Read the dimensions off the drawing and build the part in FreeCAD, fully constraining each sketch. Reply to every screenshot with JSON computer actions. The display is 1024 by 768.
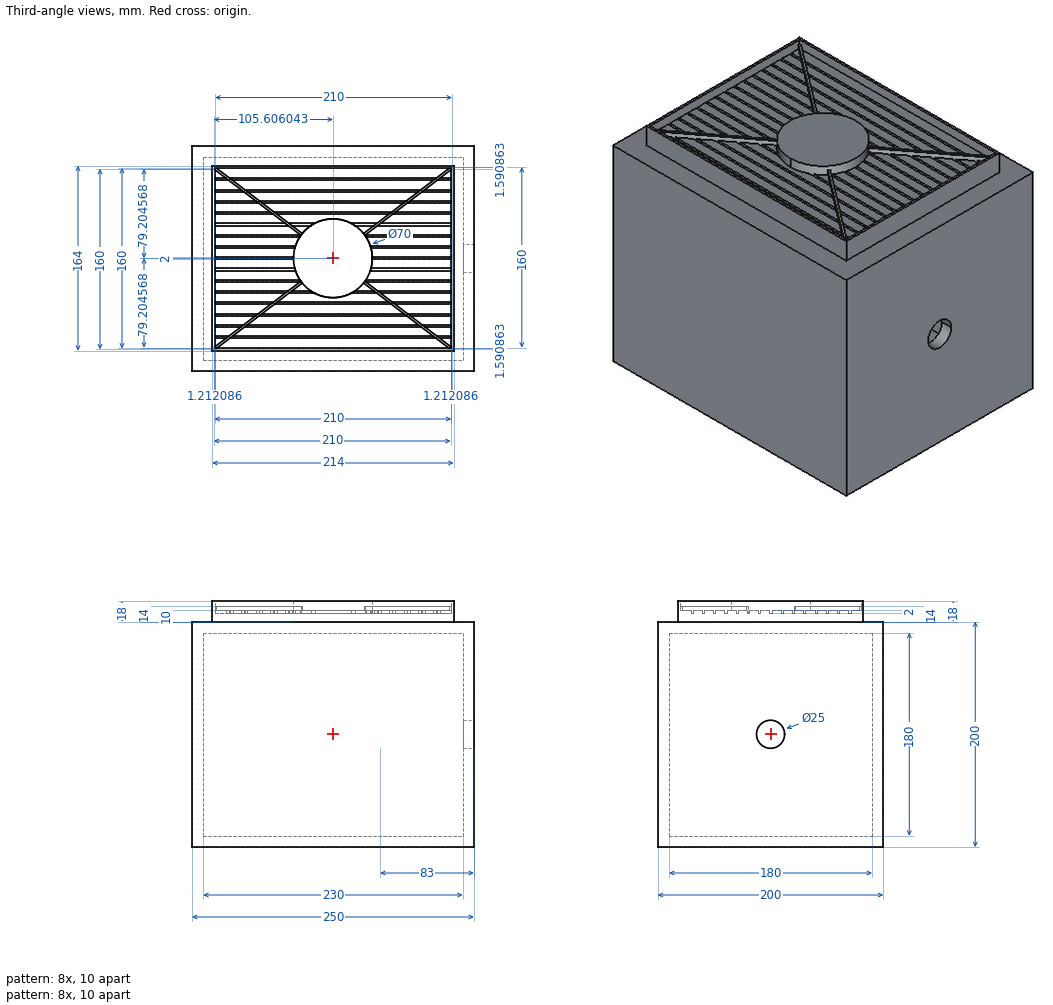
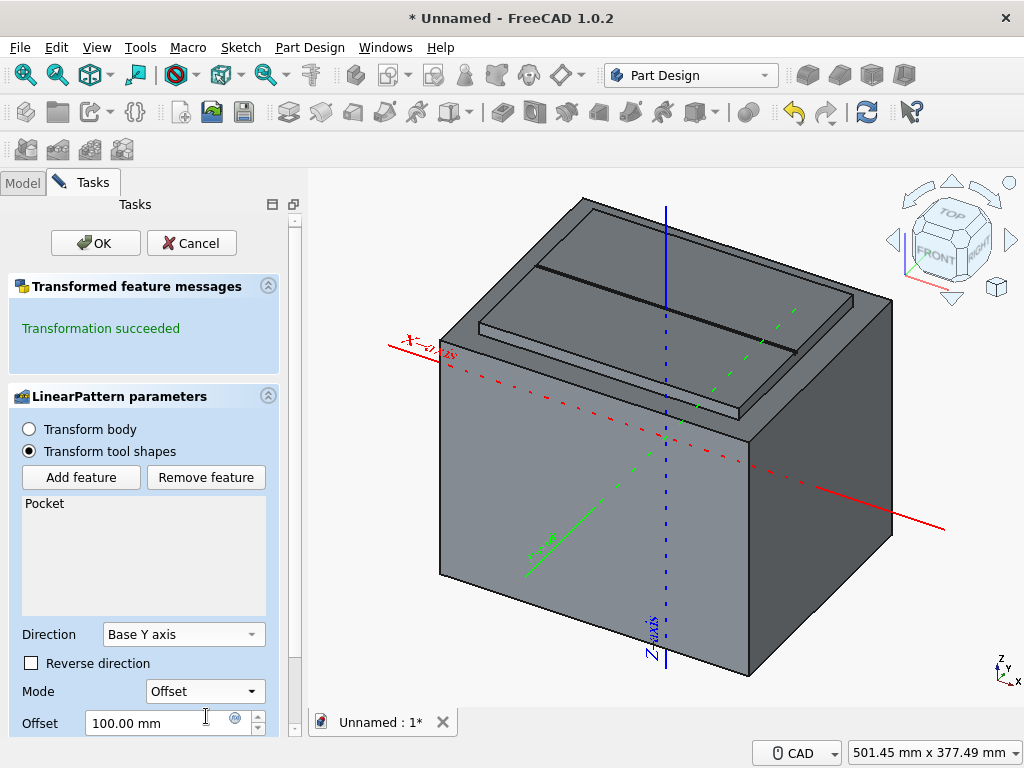
{"action": "triple_click", "coordinate": [168, 723]}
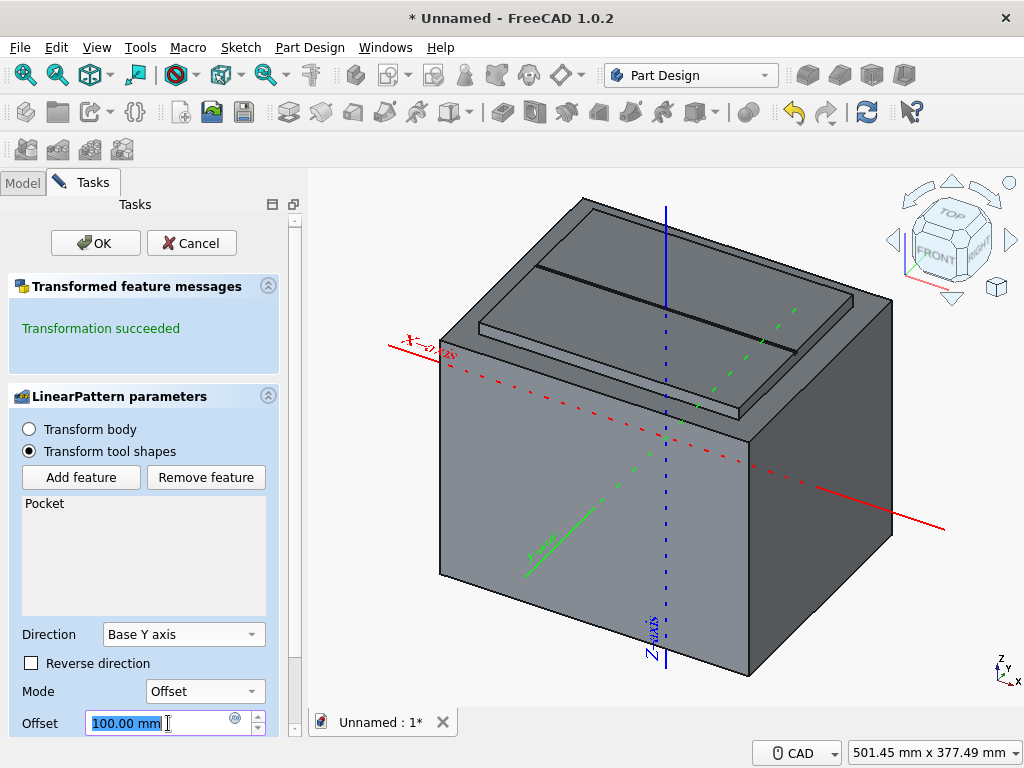
{"action": "type", "text": "10"}
{"action": "key", "text": "Tab"}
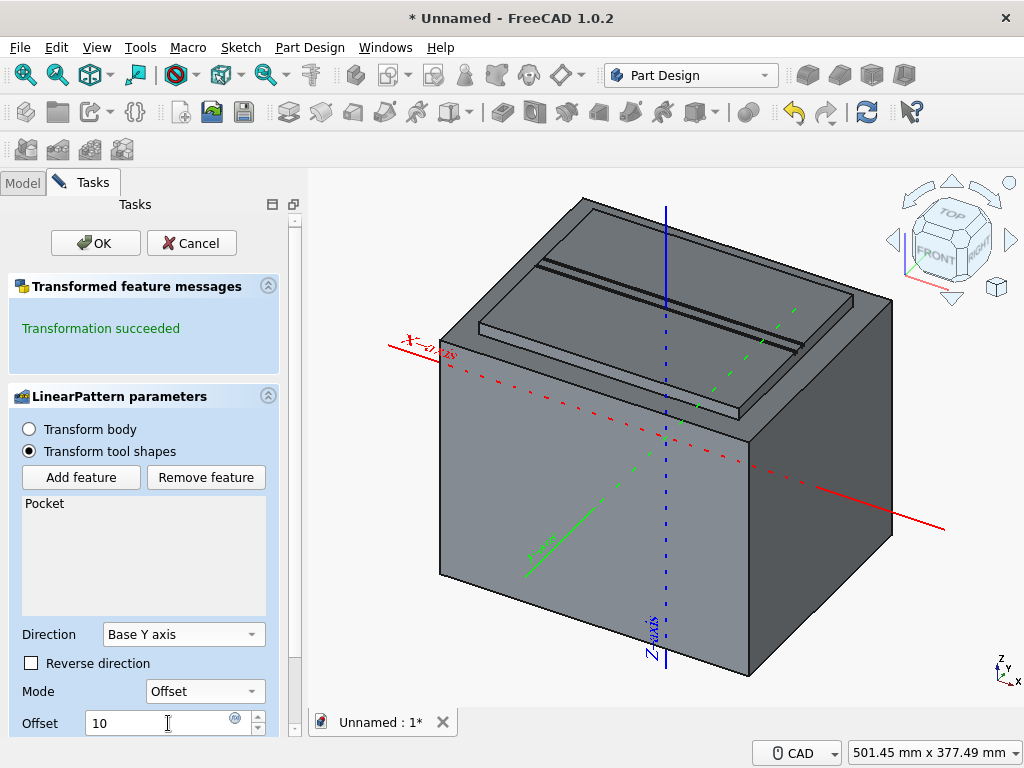
{"action": "scroll", "coordinate": [295, 475], "scroll_direction": "down", "scroll_amount": 2}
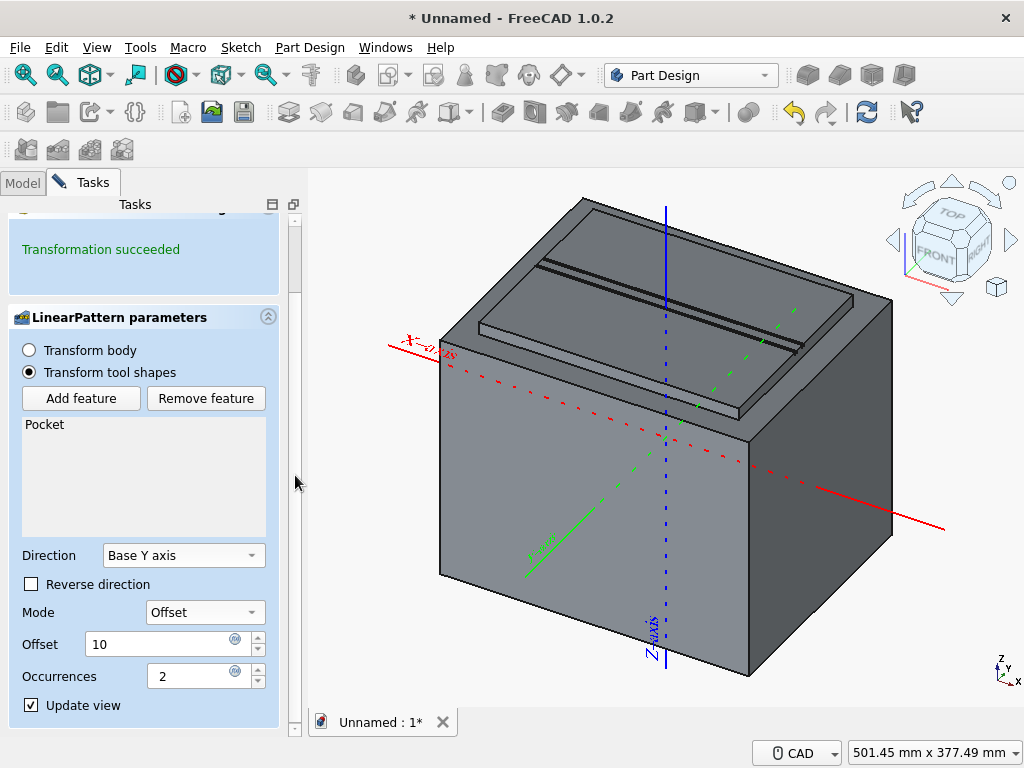
{"action": "triple_click", "coordinate": [198, 676]}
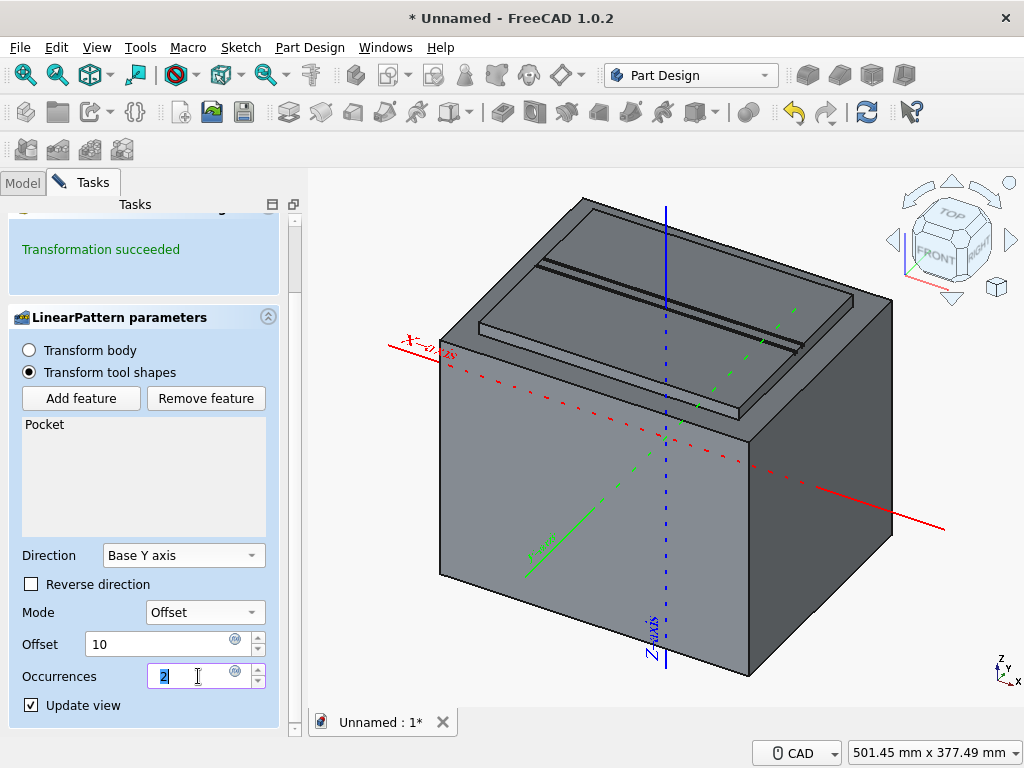
{"action": "type", "text": "8"}
{"action": "key", "text": "Tab"}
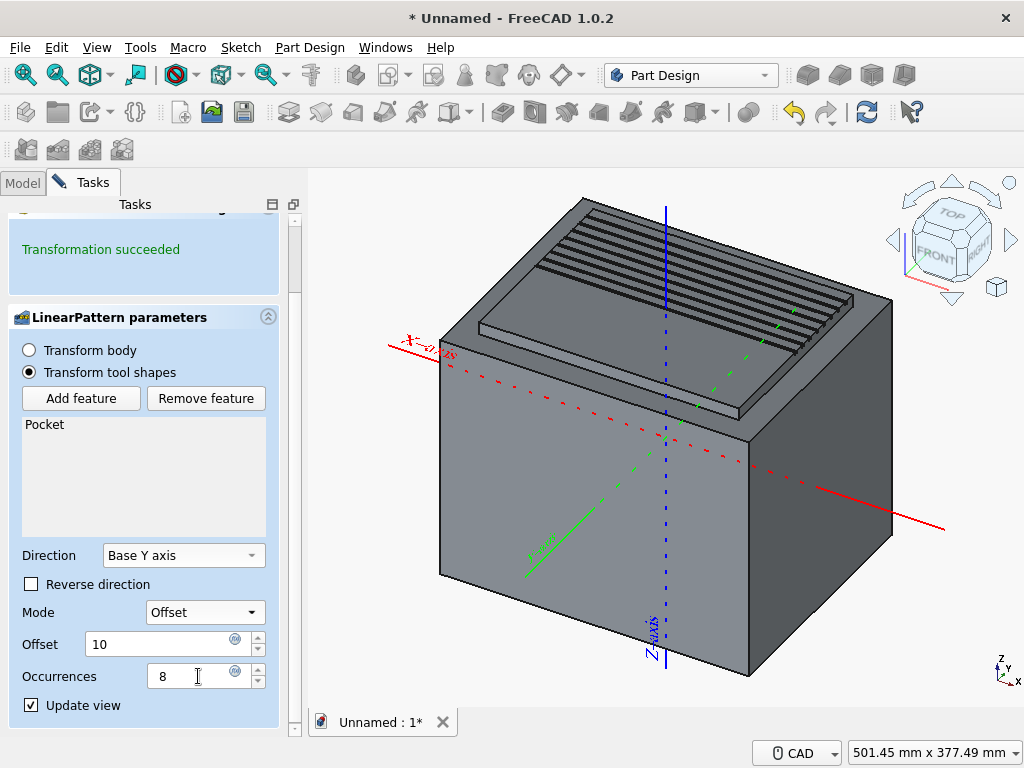
{"action": "scroll", "coordinate": [295, 475], "scroll_direction": "up", "scroll_amount": 3}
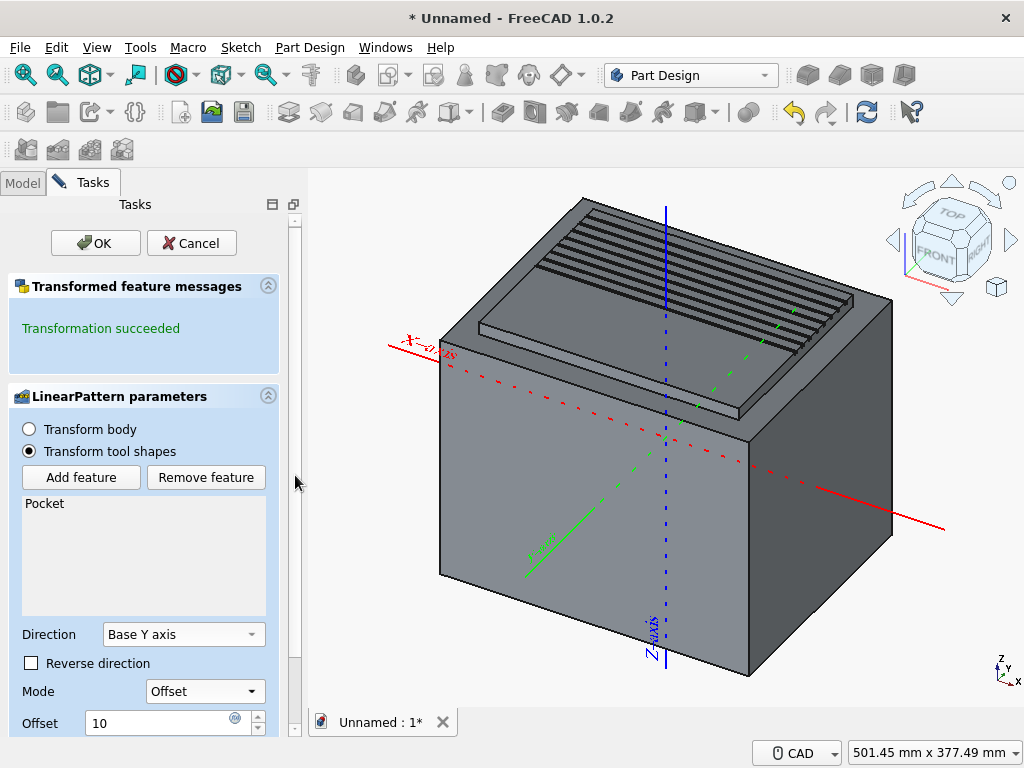
{"action": "left_click", "coordinate": [96, 243]}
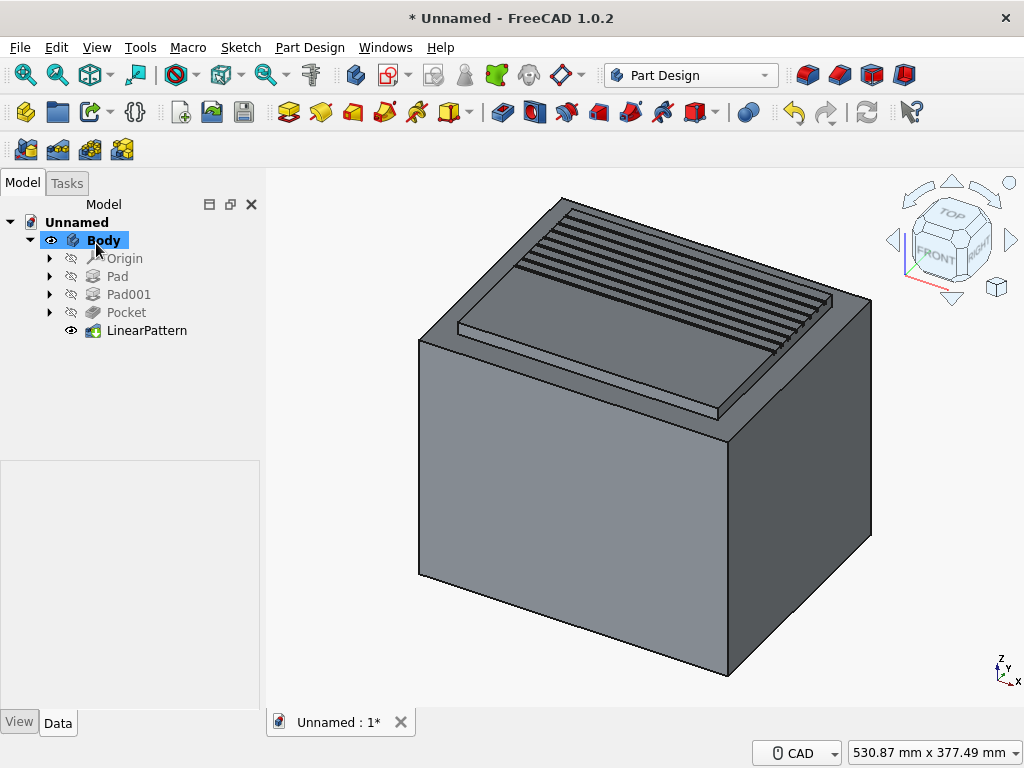
{"action": "left_click", "coordinate": [116, 312]}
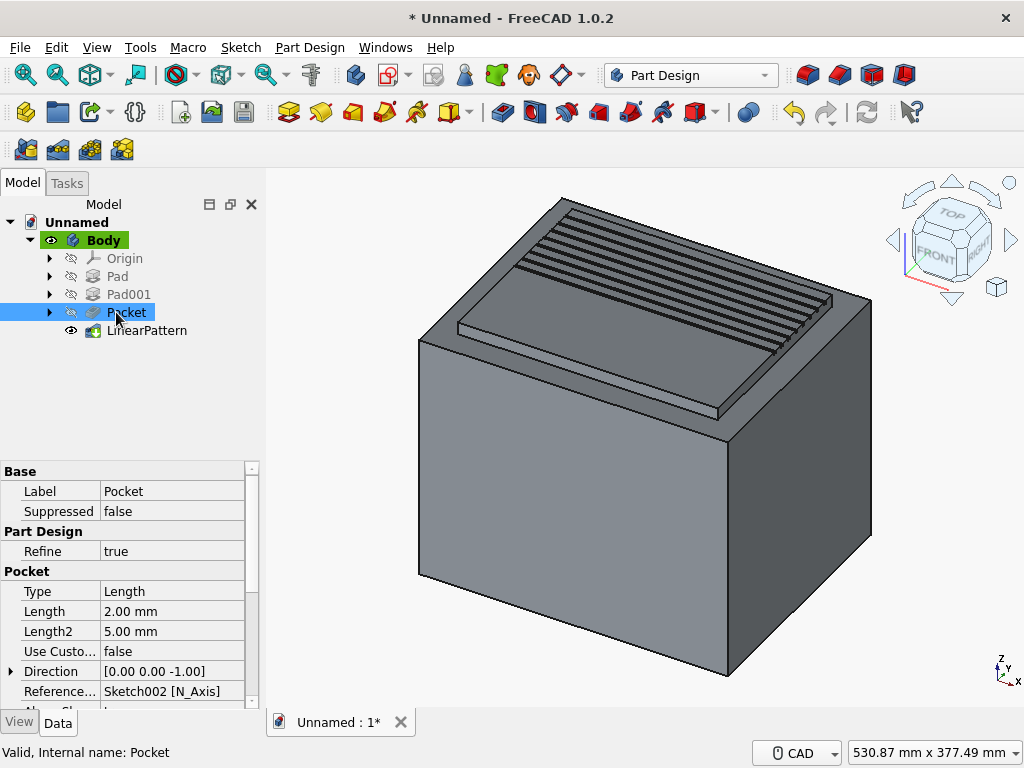
{"action": "left_click", "coordinate": [58, 150]}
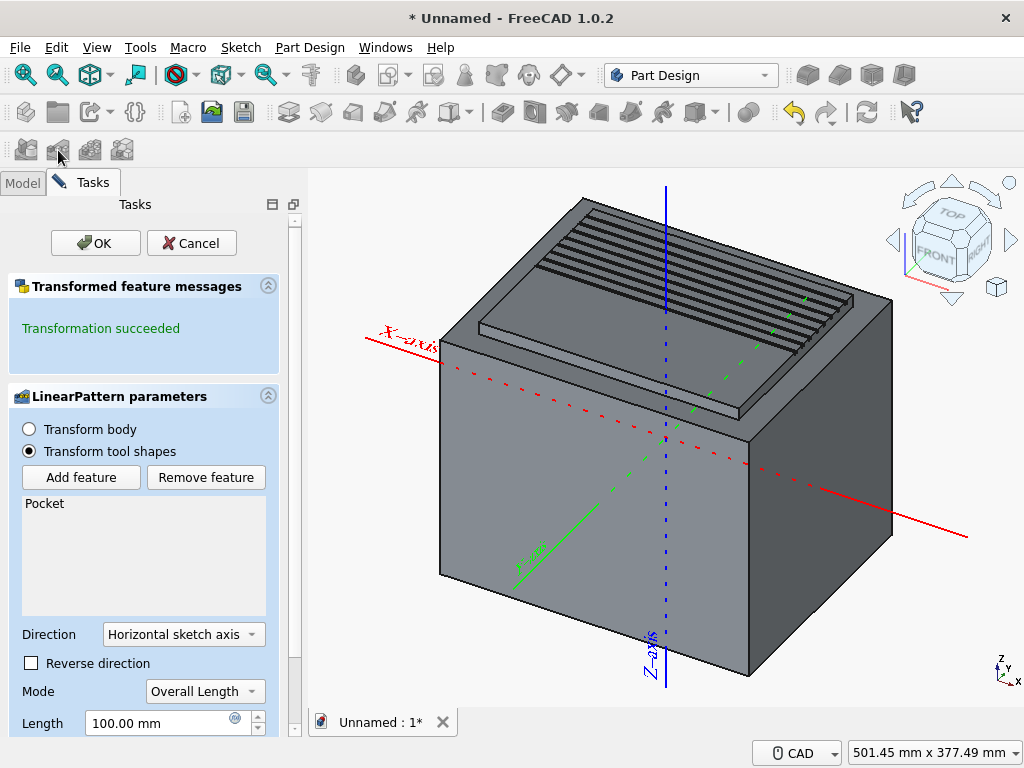
{"action": "left_click", "coordinate": [184, 634]}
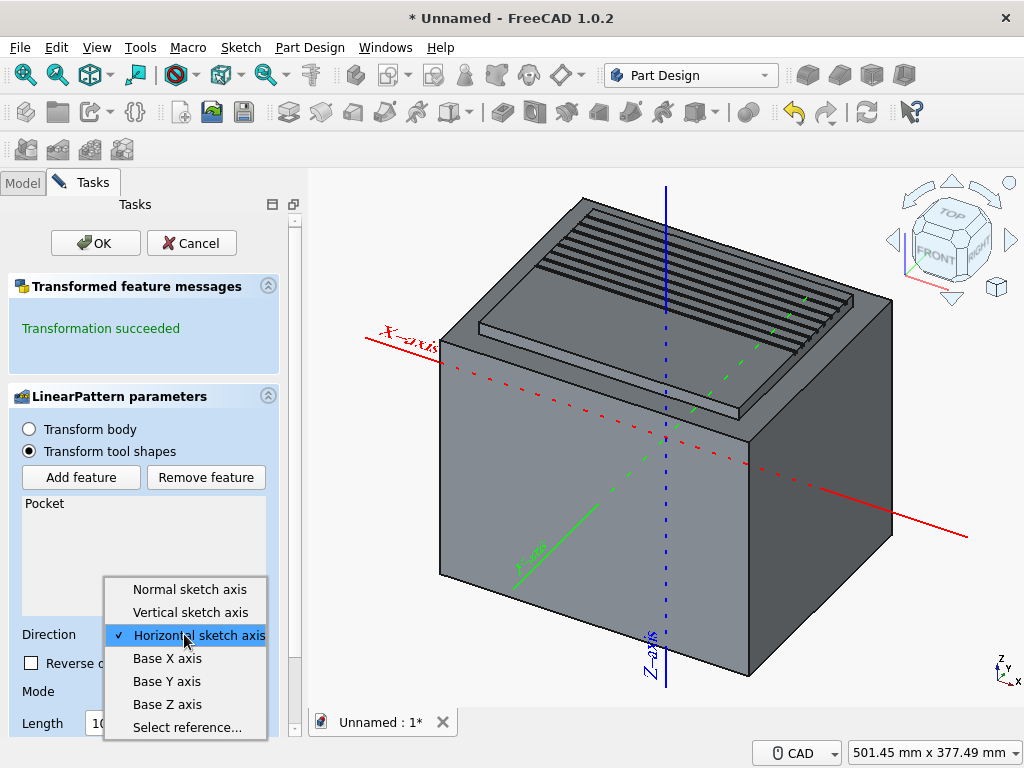
{"action": "left_click", "coordinate": [184, 682]}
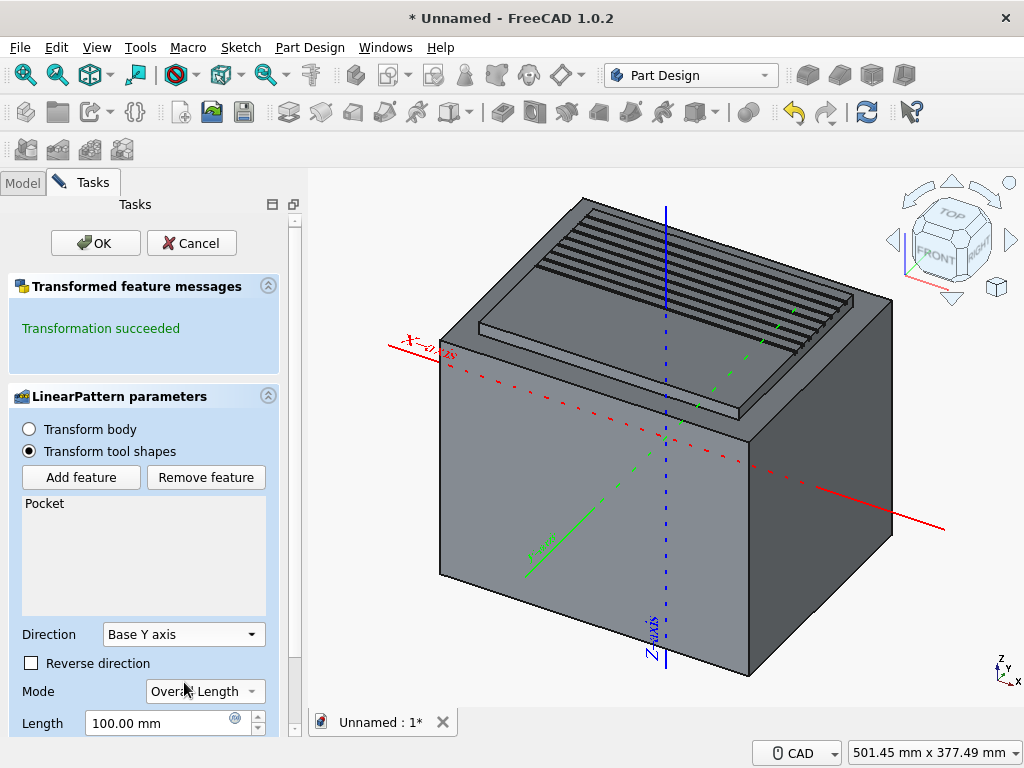
{"action": "left_click", "coordinate": [206, 692]}